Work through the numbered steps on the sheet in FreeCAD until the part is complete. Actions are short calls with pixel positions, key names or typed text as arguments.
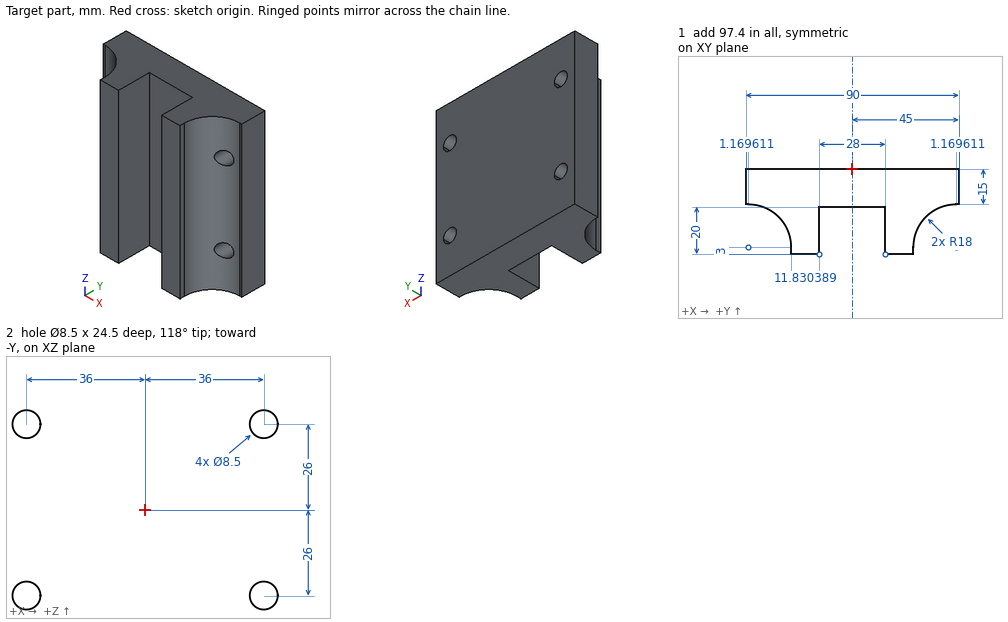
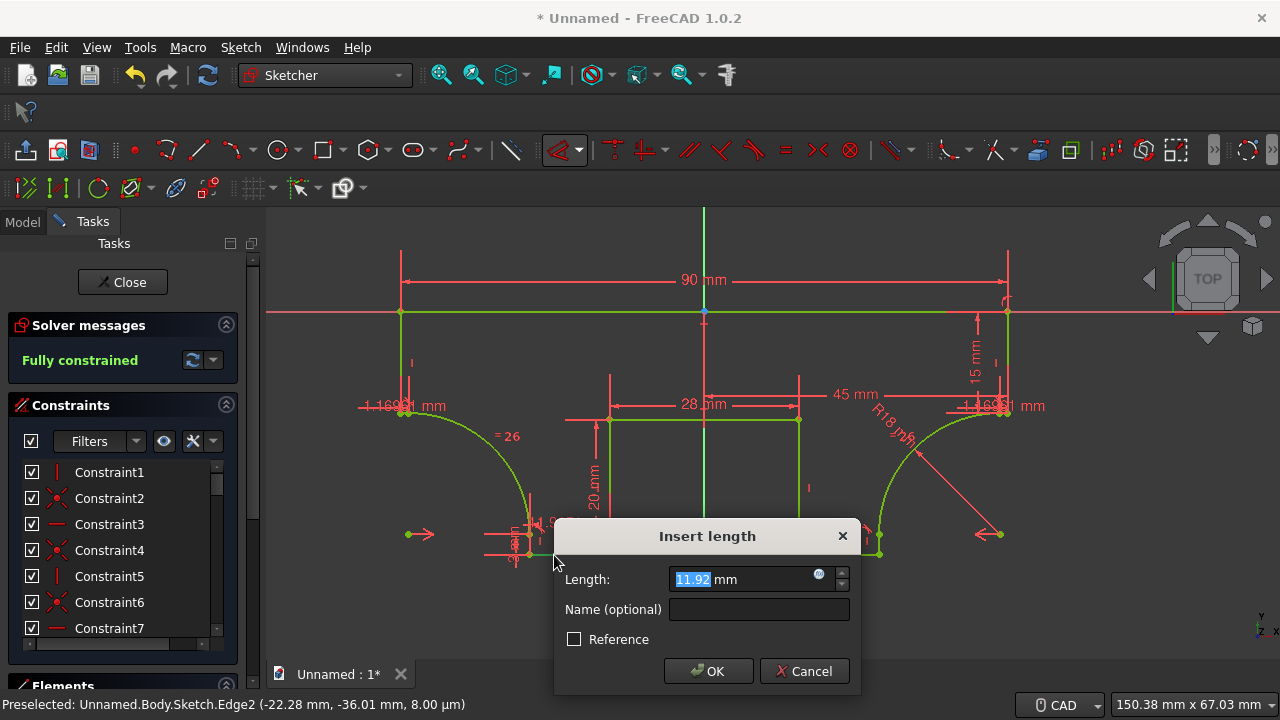
text(11.830389)
key(Return)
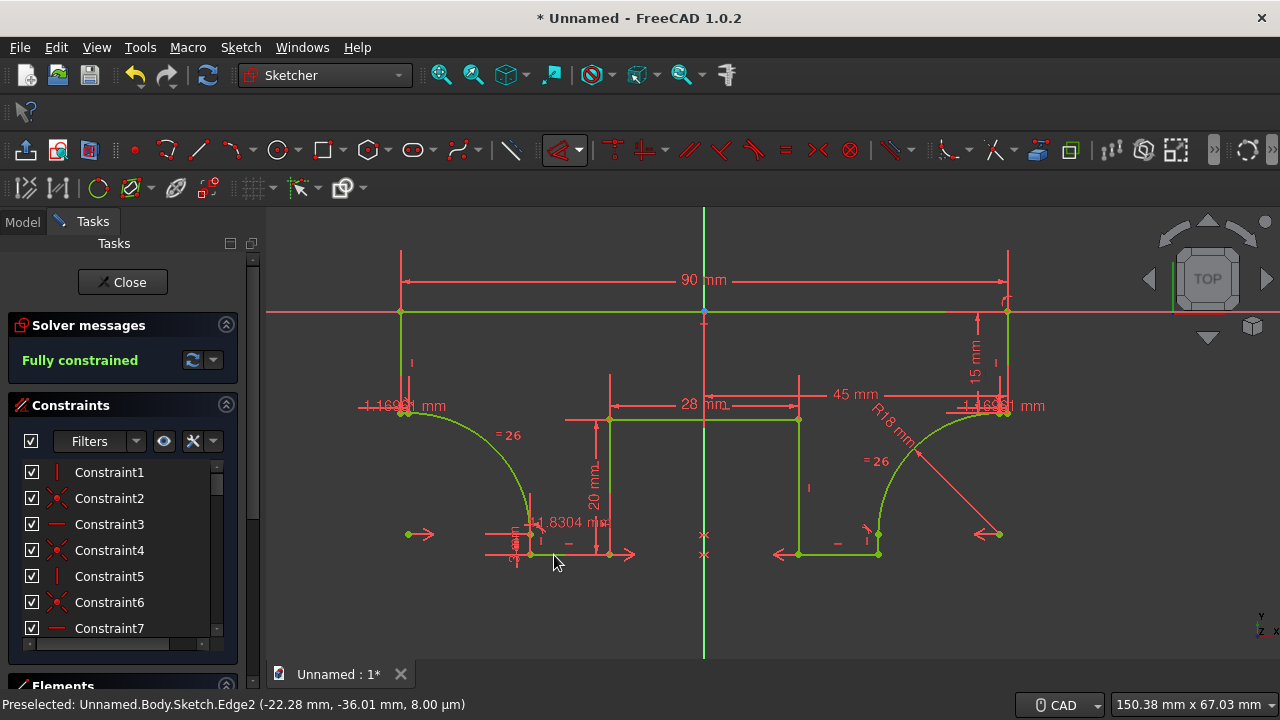
click(123, 282)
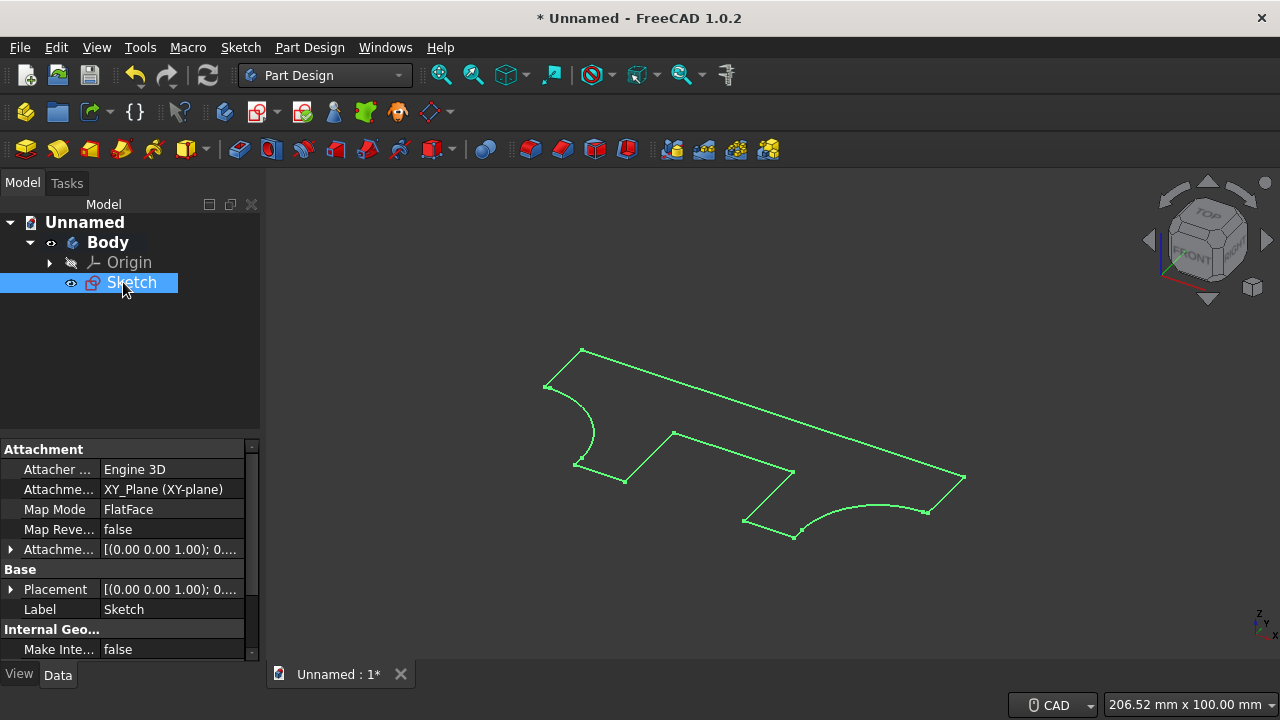
click(26, 150)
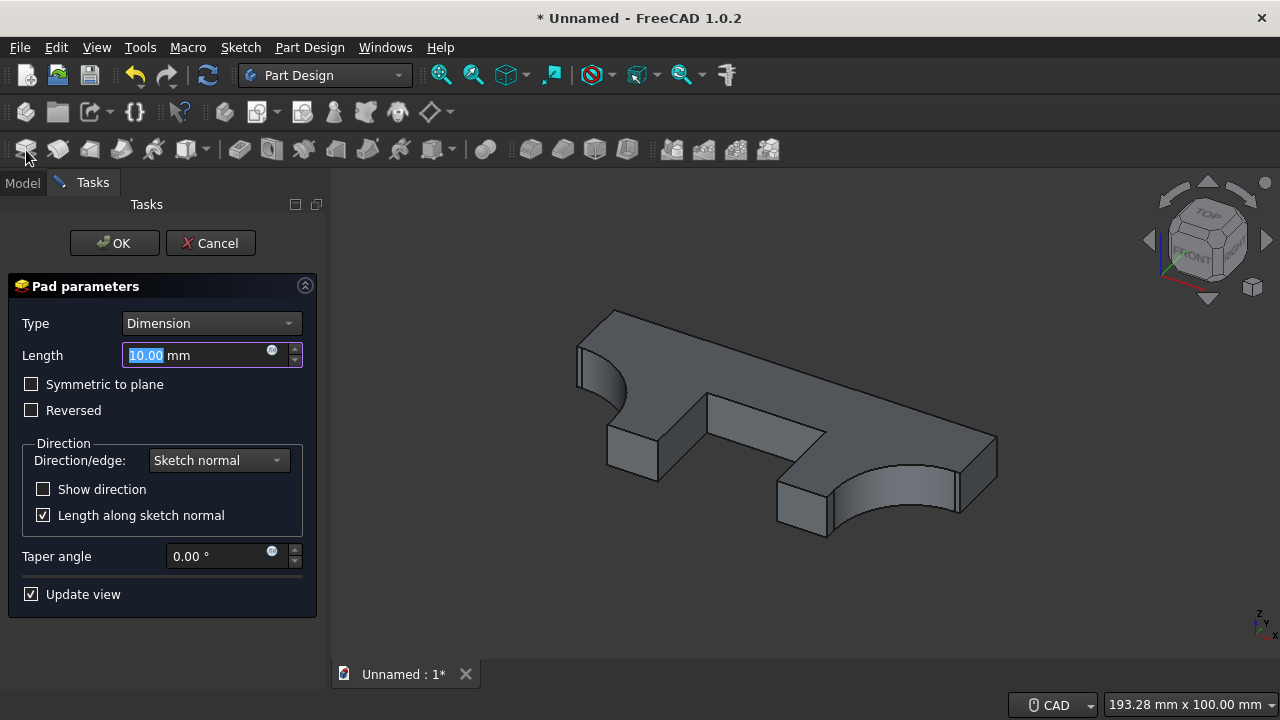
text(97.4)
key(Tab)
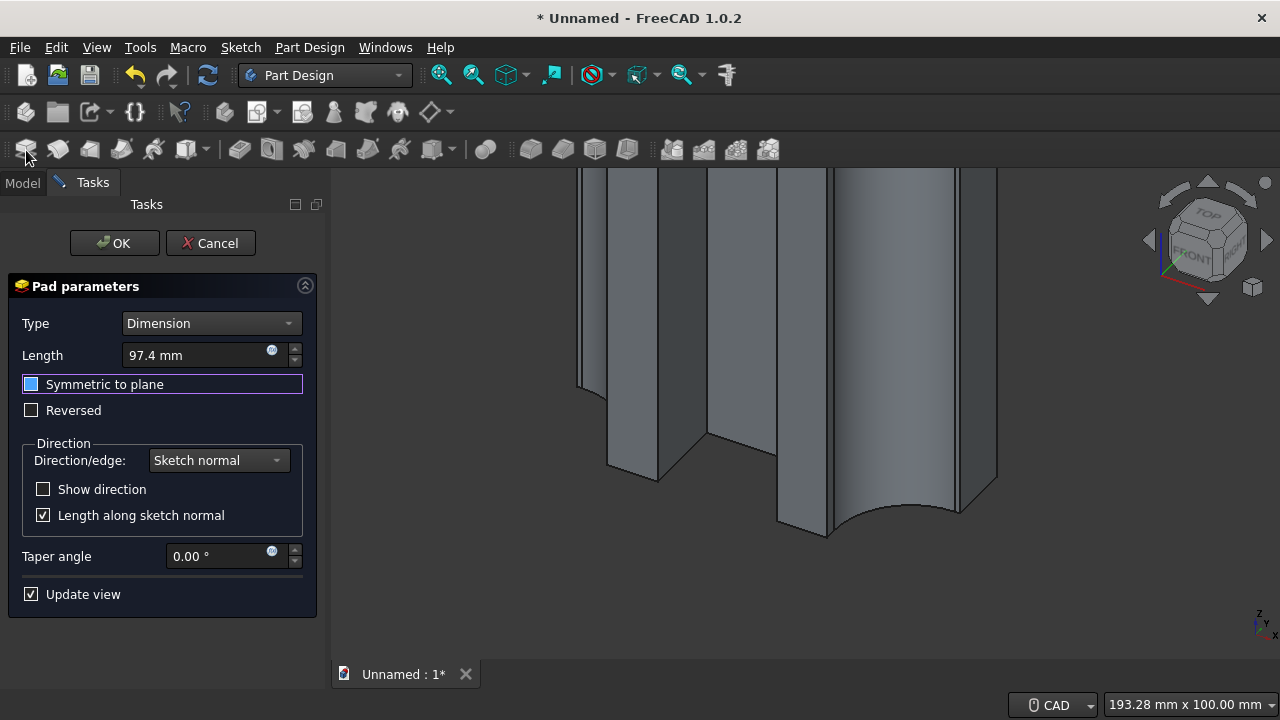
click(30, 384)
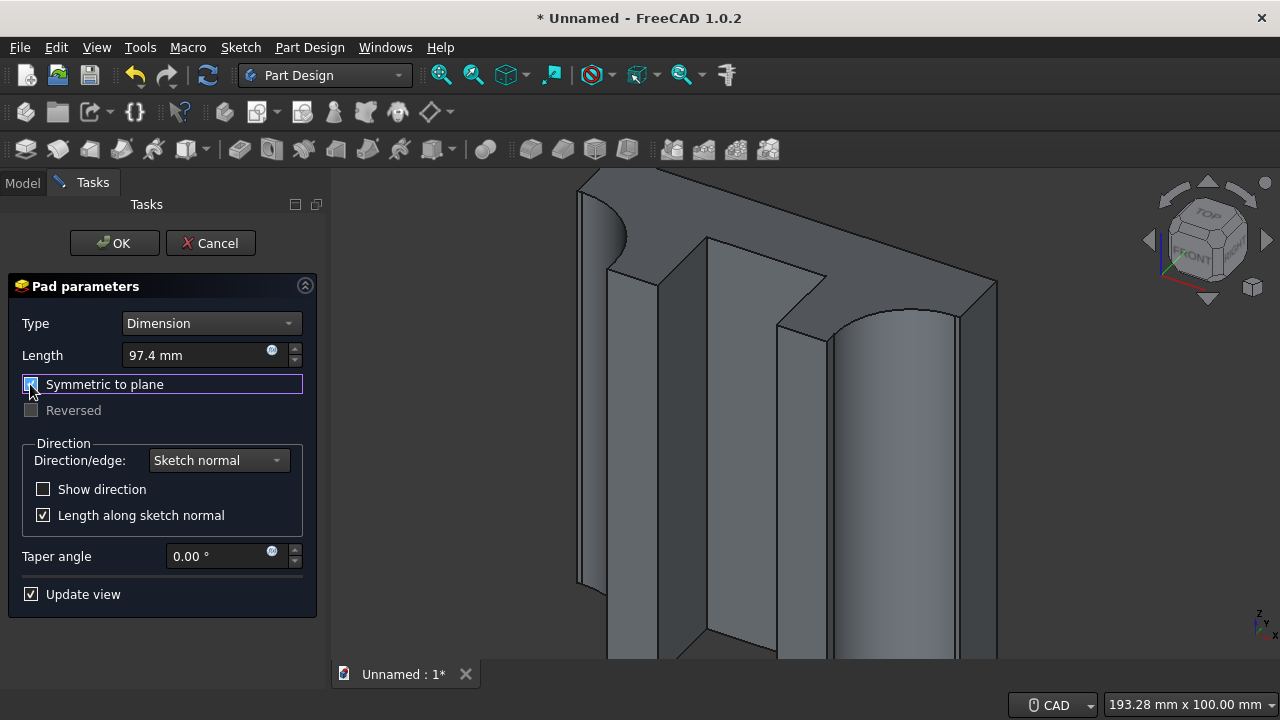
click(115, 243)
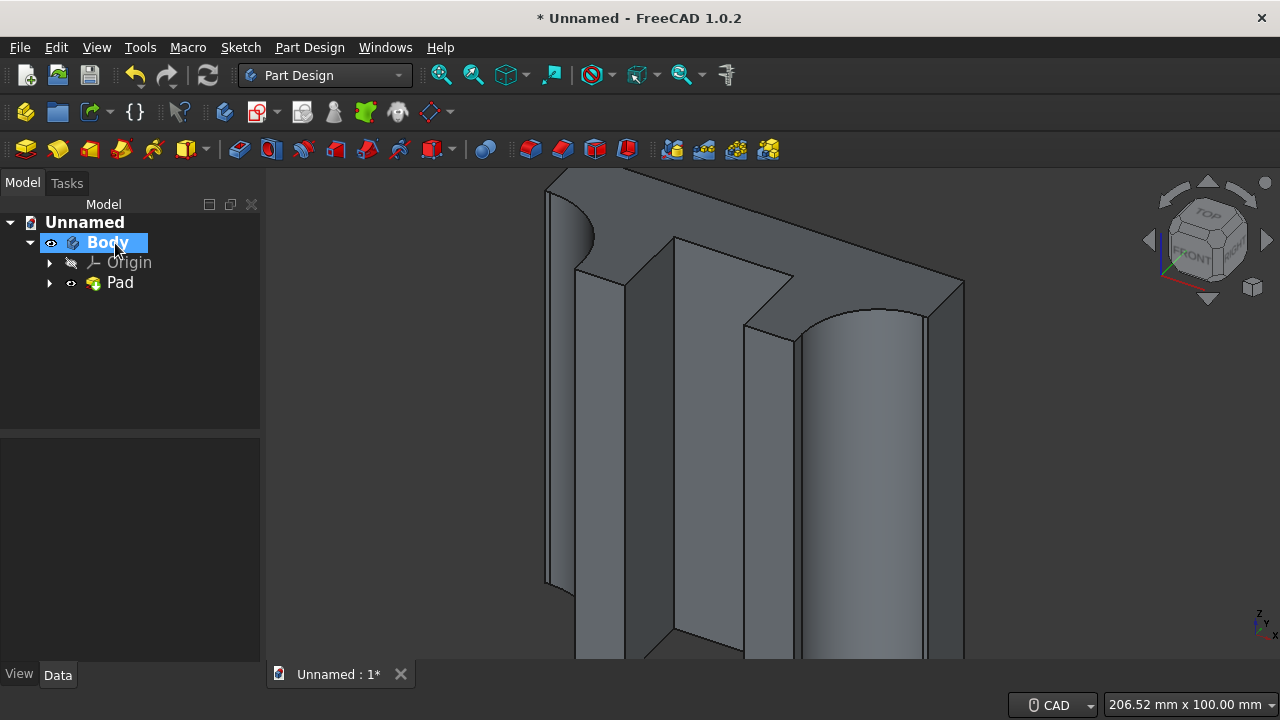
click(442, 76)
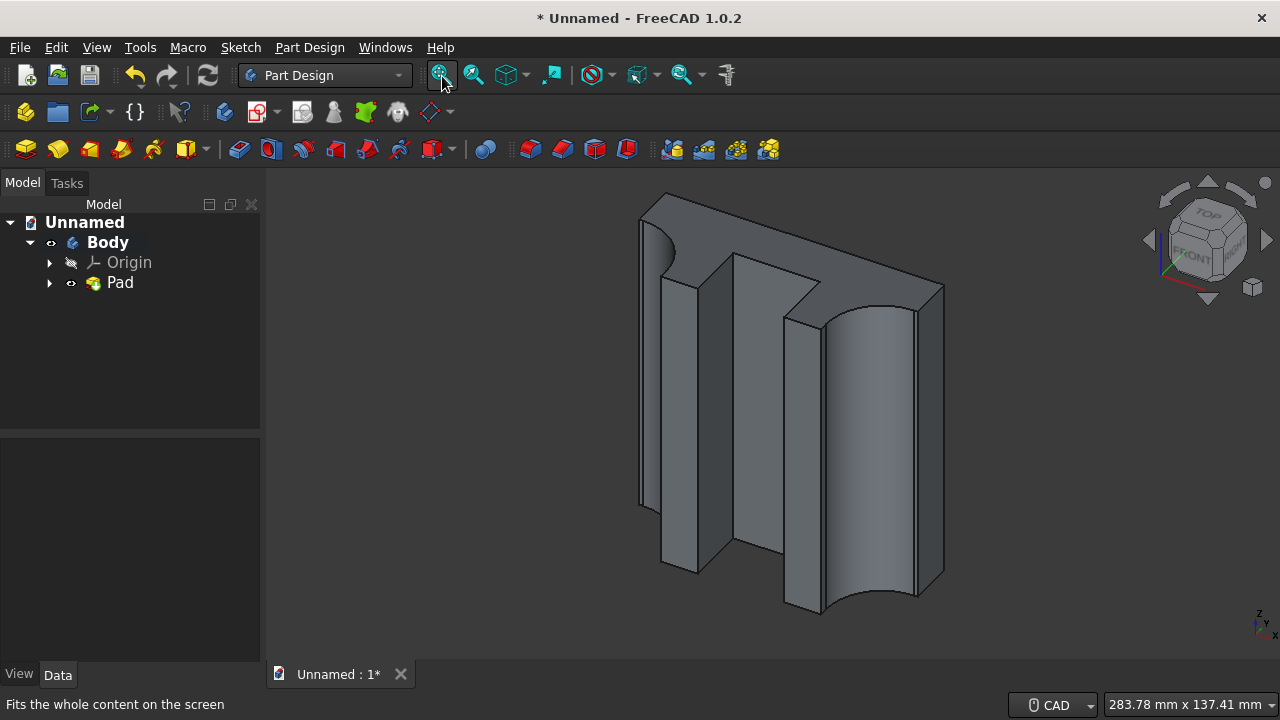
click(258, 112)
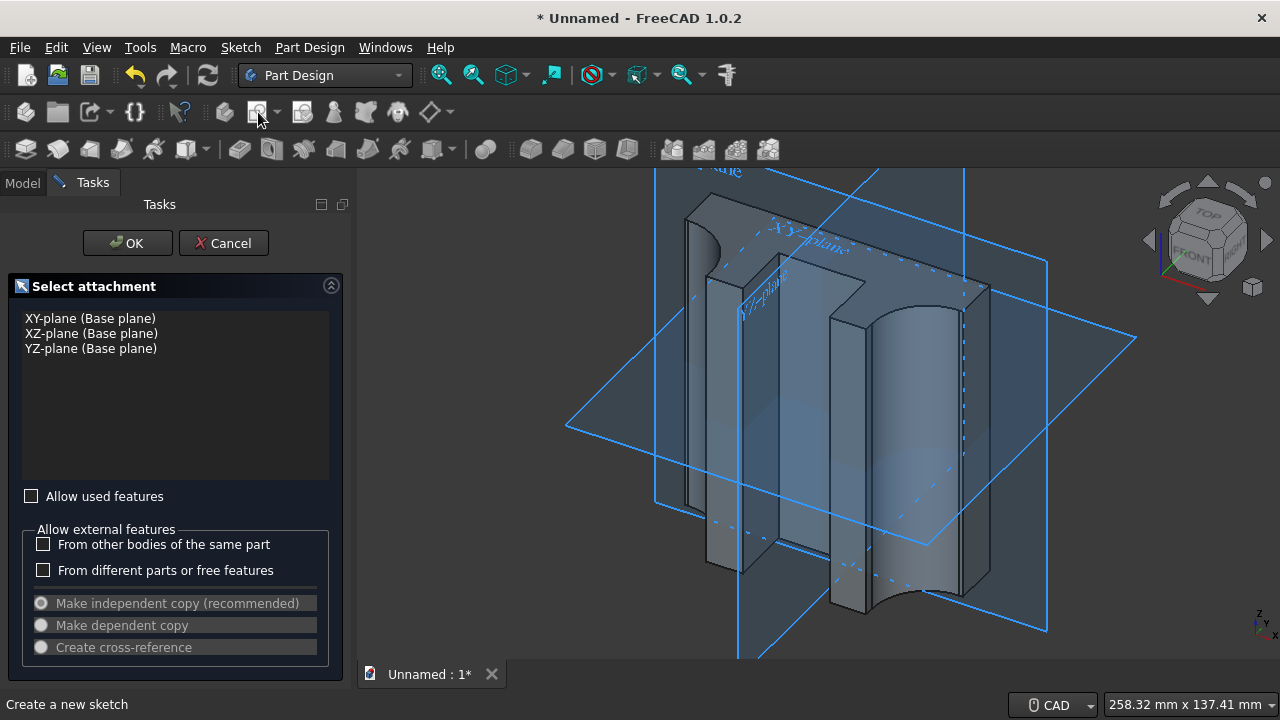
click(82, 334)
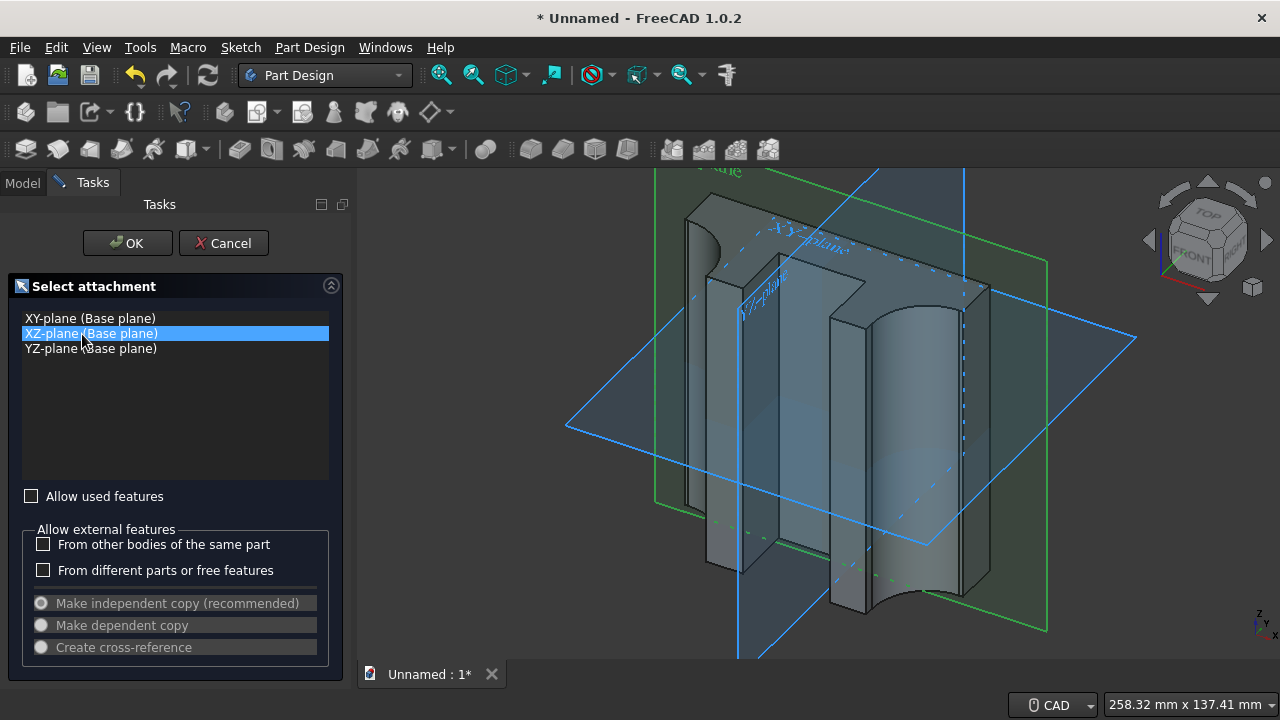
click(128, 243)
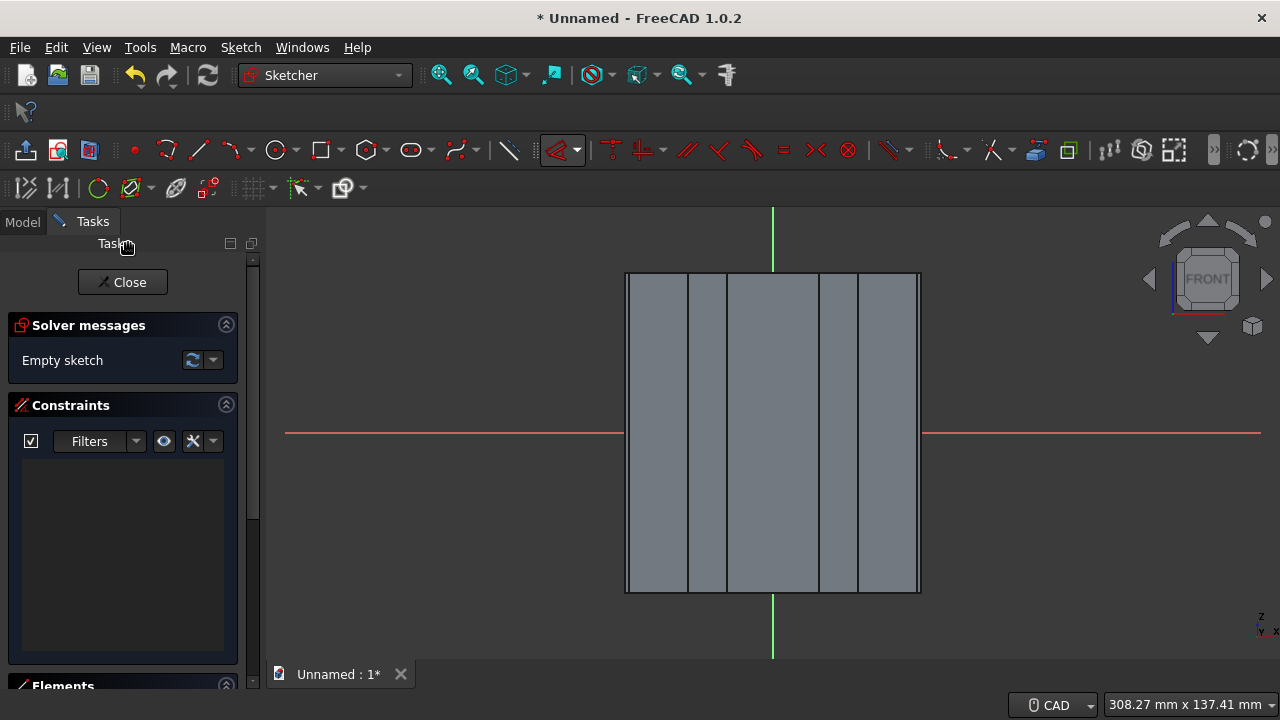
key(q)
key(s)